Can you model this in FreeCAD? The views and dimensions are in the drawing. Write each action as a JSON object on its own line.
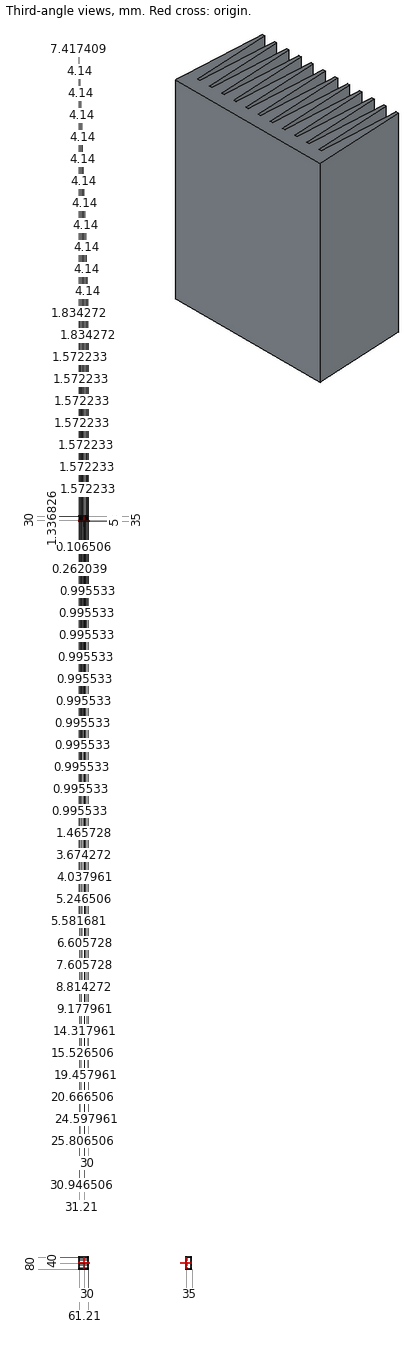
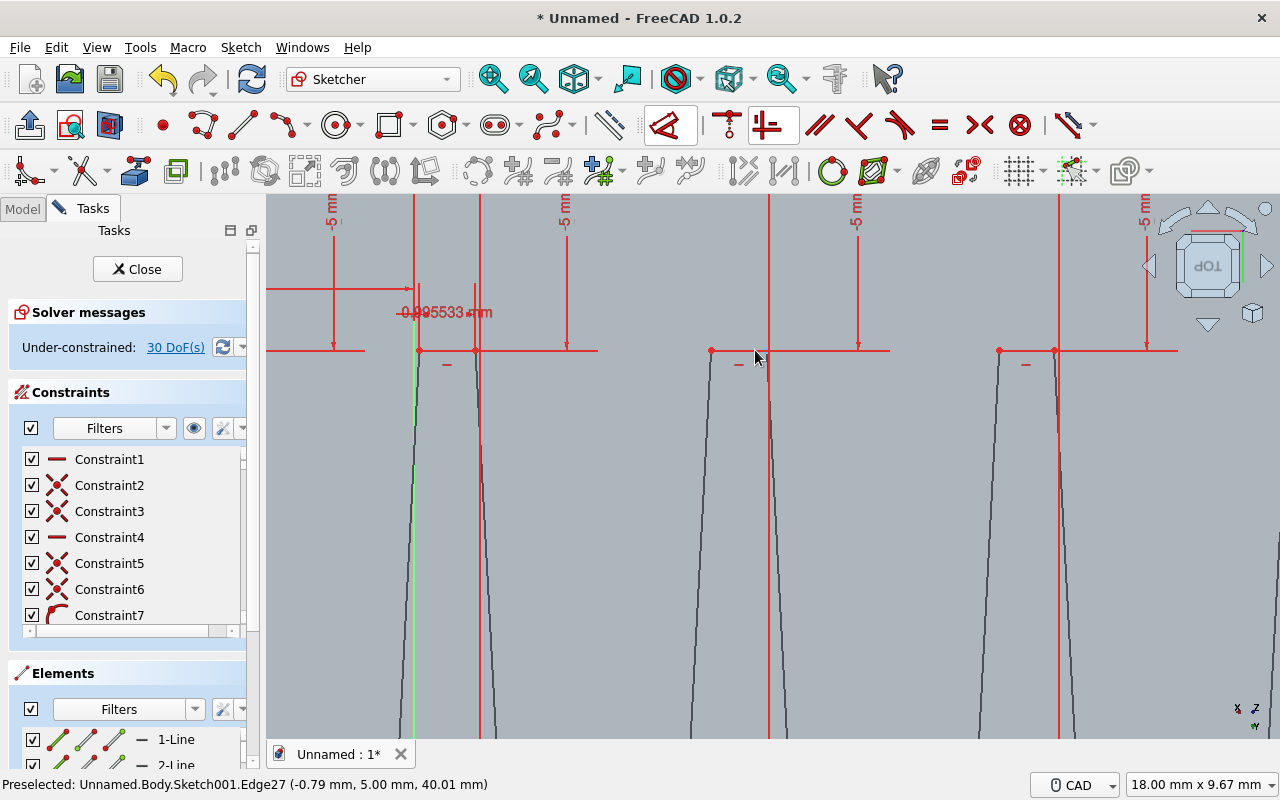
{"action": "left_click", "coordinate": [750, 351]}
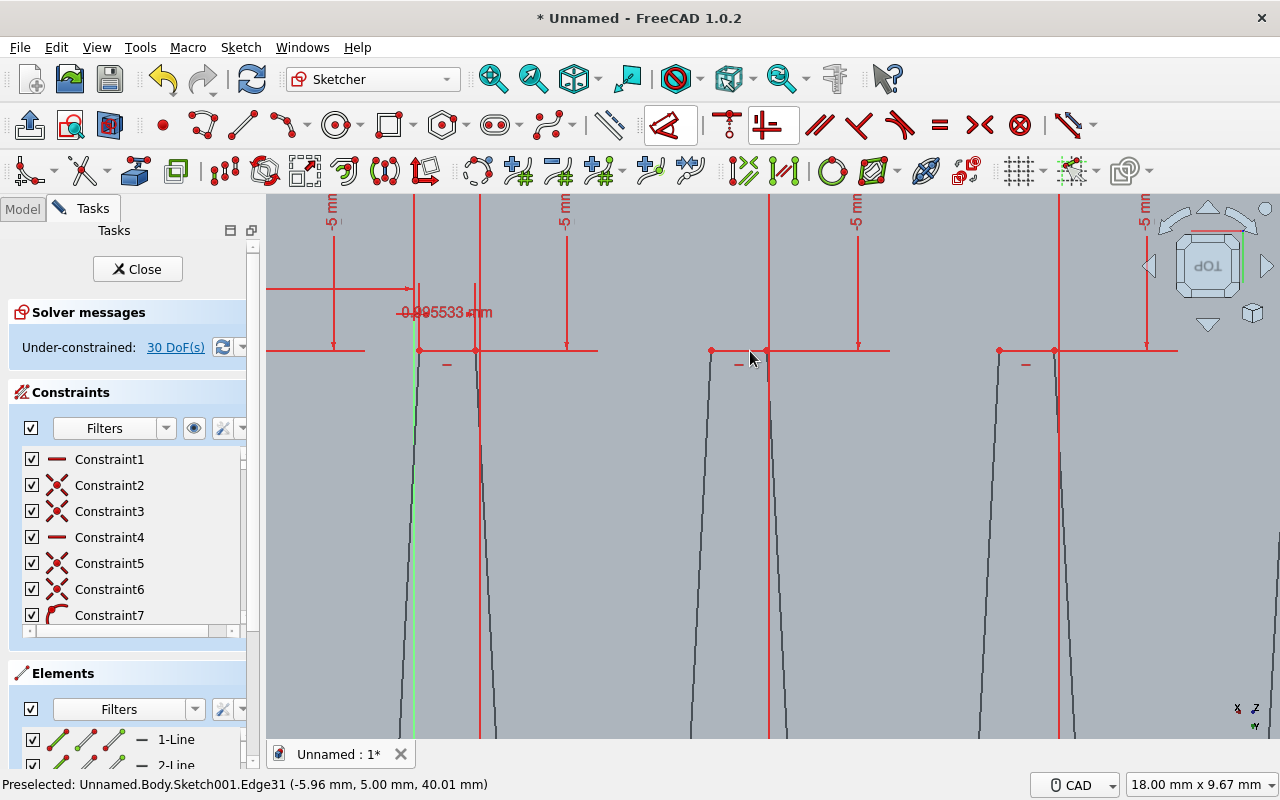
{"action": "left_click", "coordinate": [692, 126]}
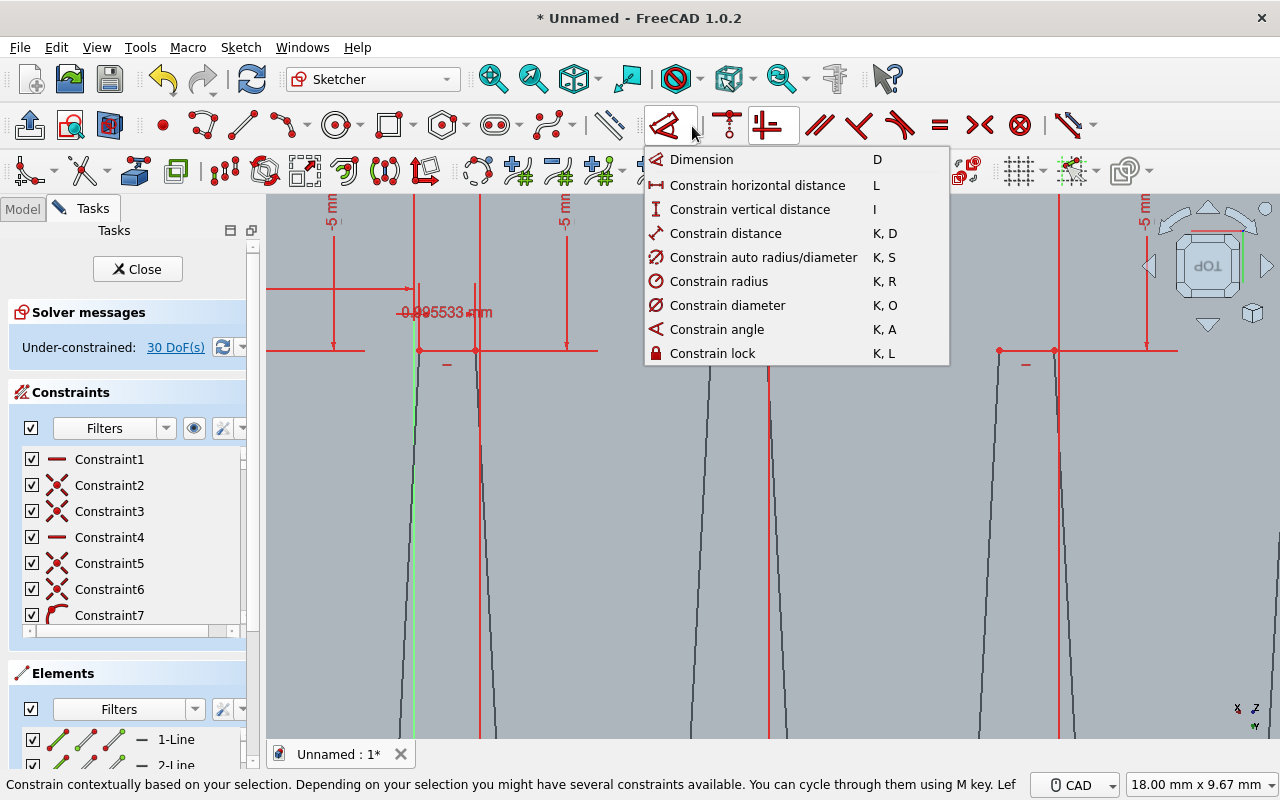
{"action": "left_click", "coordinate": [797, 185]}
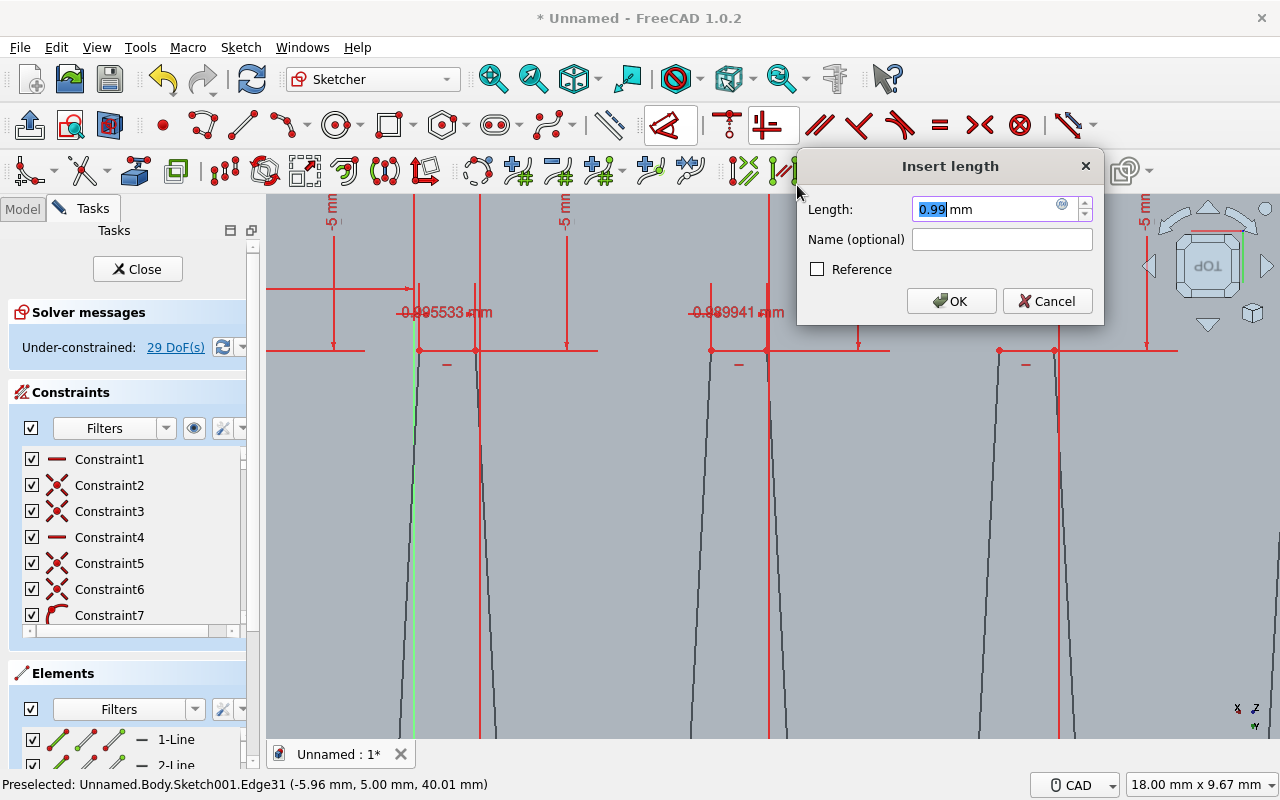
{"action": "type", "text": "0.995533"}
{"action": "key", "text": "Return"}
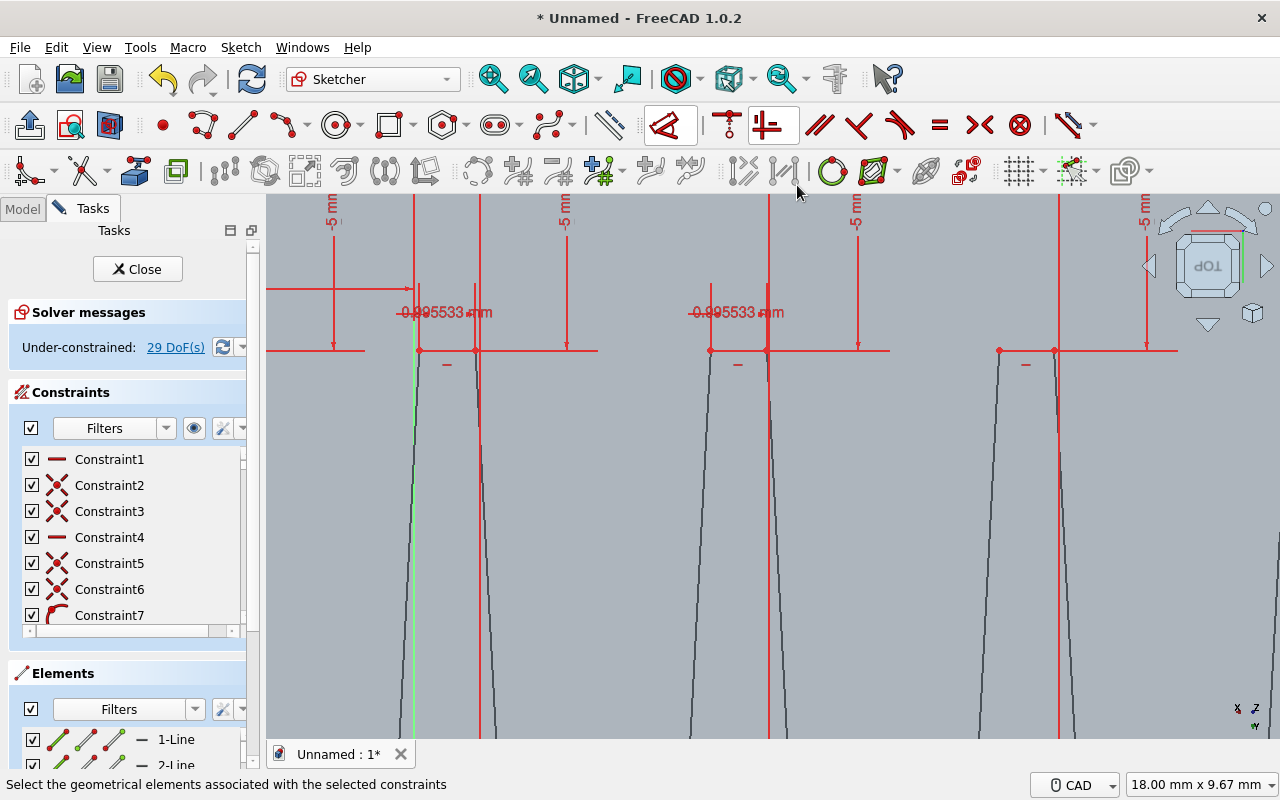
{"action": "left_click", "coordinate": [1038, 351]}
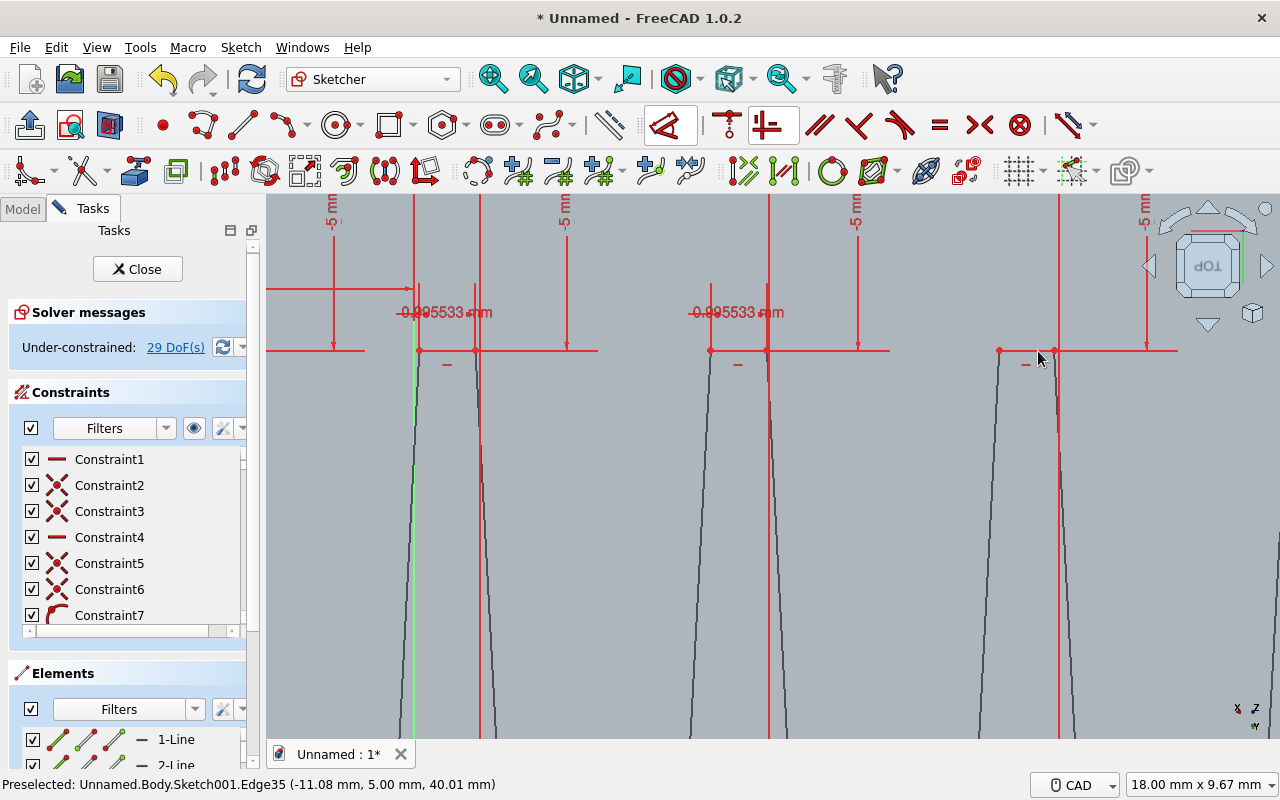
{"action": "key", "text": "l"}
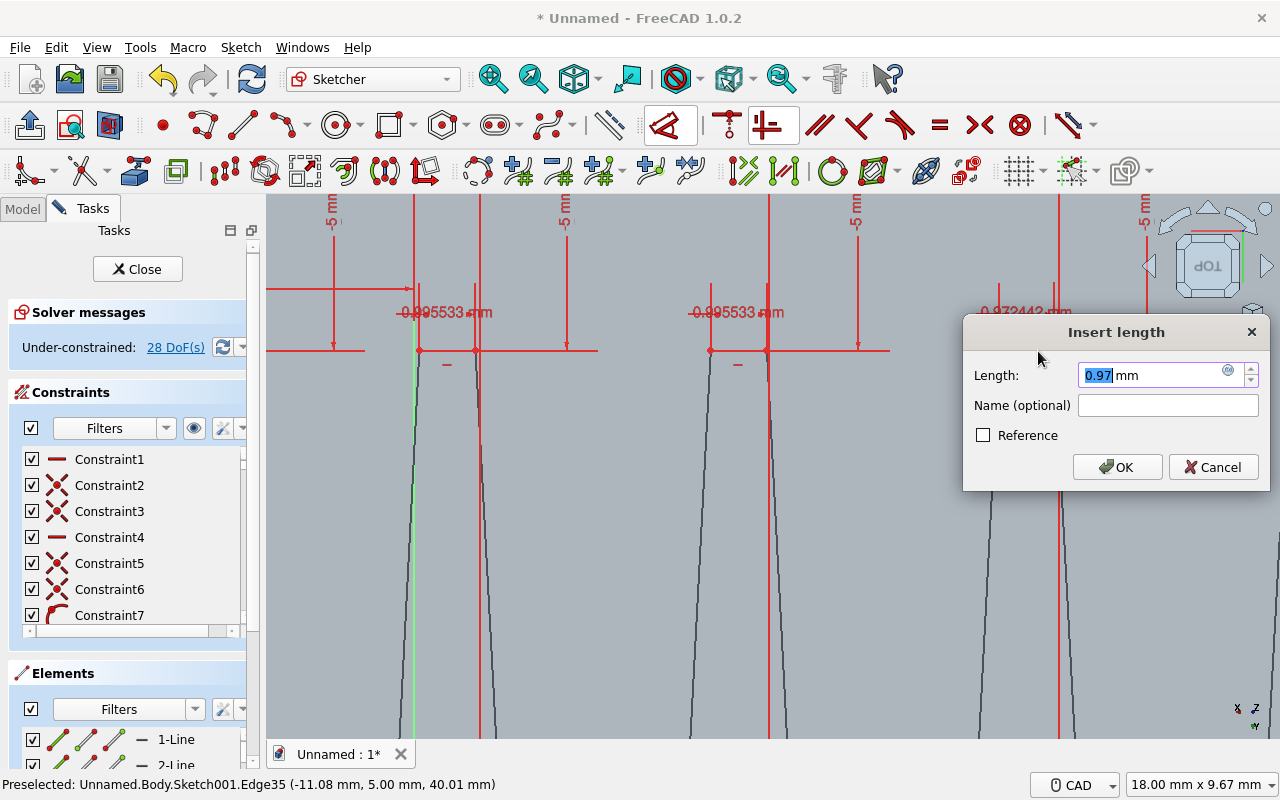
{"action": "type", "text": "0.995533"}
{"action": "key", "text": "Return"}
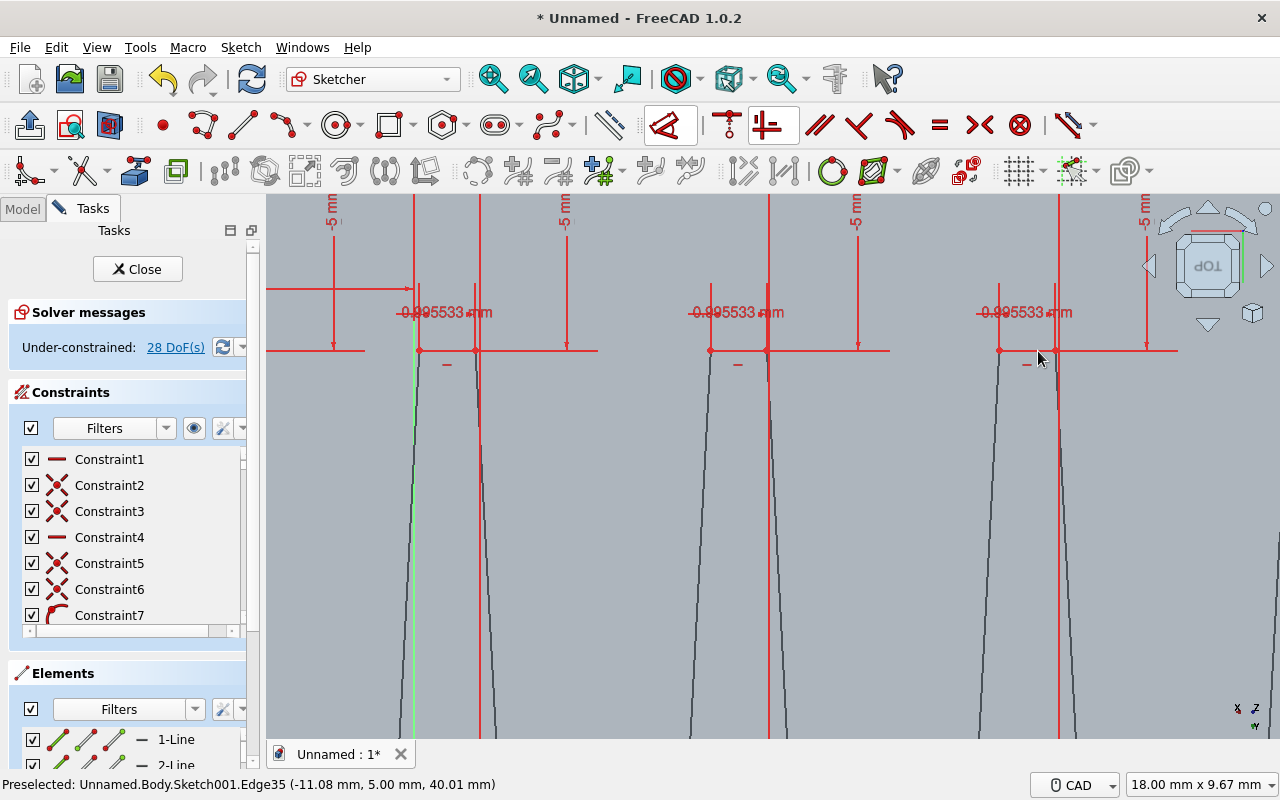
{"action": "scroll", "coordinate": [755, 350], "scroll_direction": "down", "scroll_amount": 9}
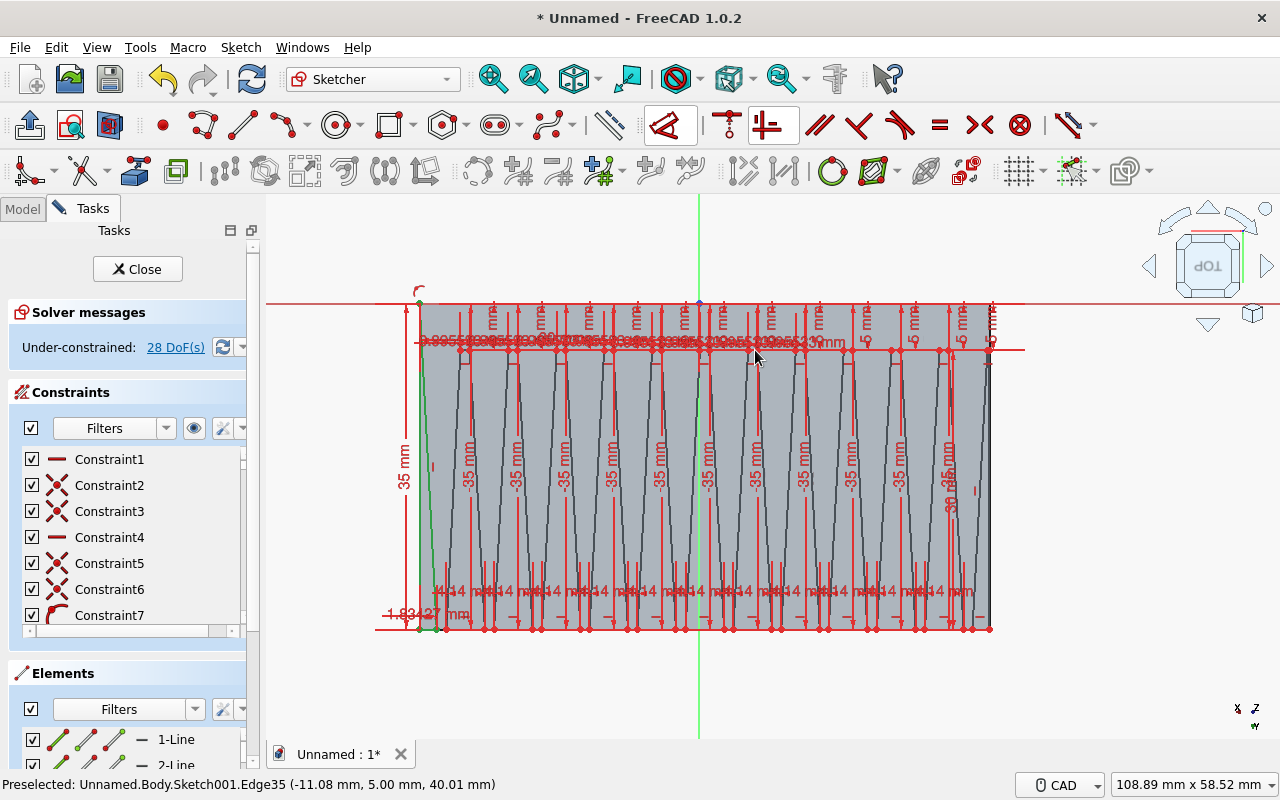
{"action": "scroll", "coordinate": [850, 350], "scroll_direction": "up", "scroll_amount": 9}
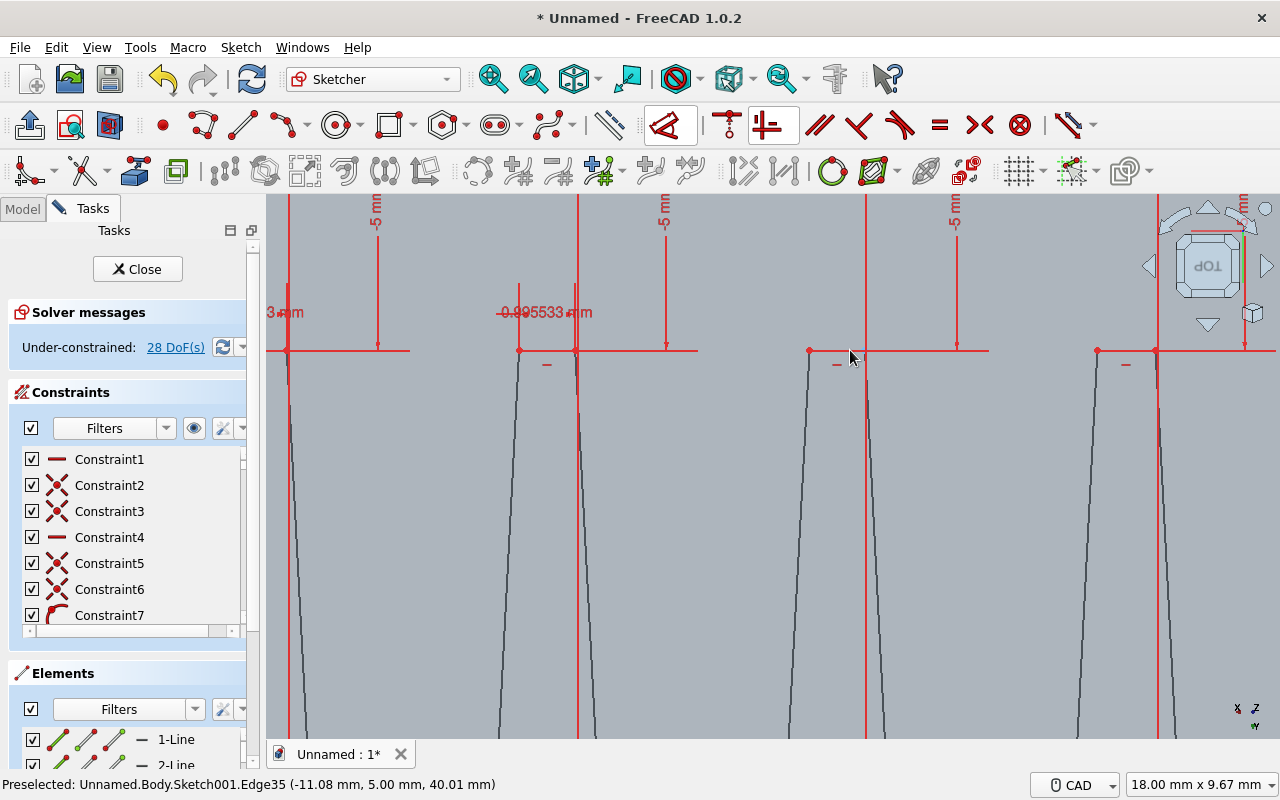
{"action": "left_click", "coordinate": [848, 351]}